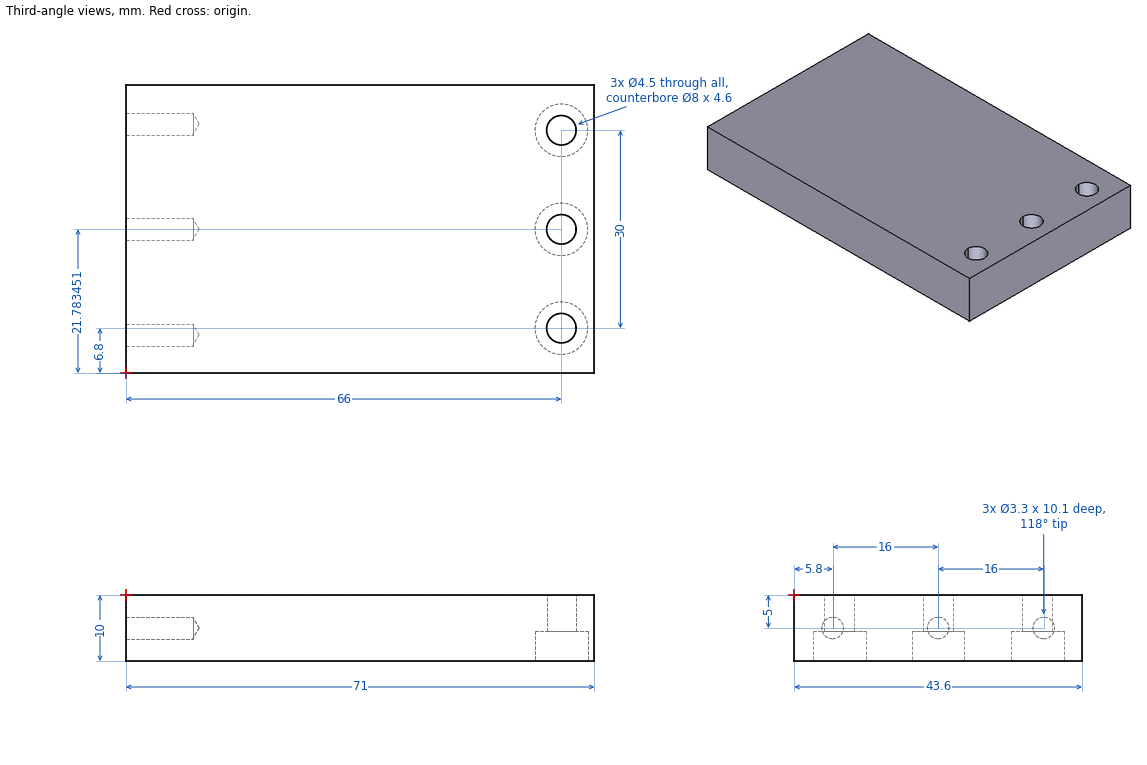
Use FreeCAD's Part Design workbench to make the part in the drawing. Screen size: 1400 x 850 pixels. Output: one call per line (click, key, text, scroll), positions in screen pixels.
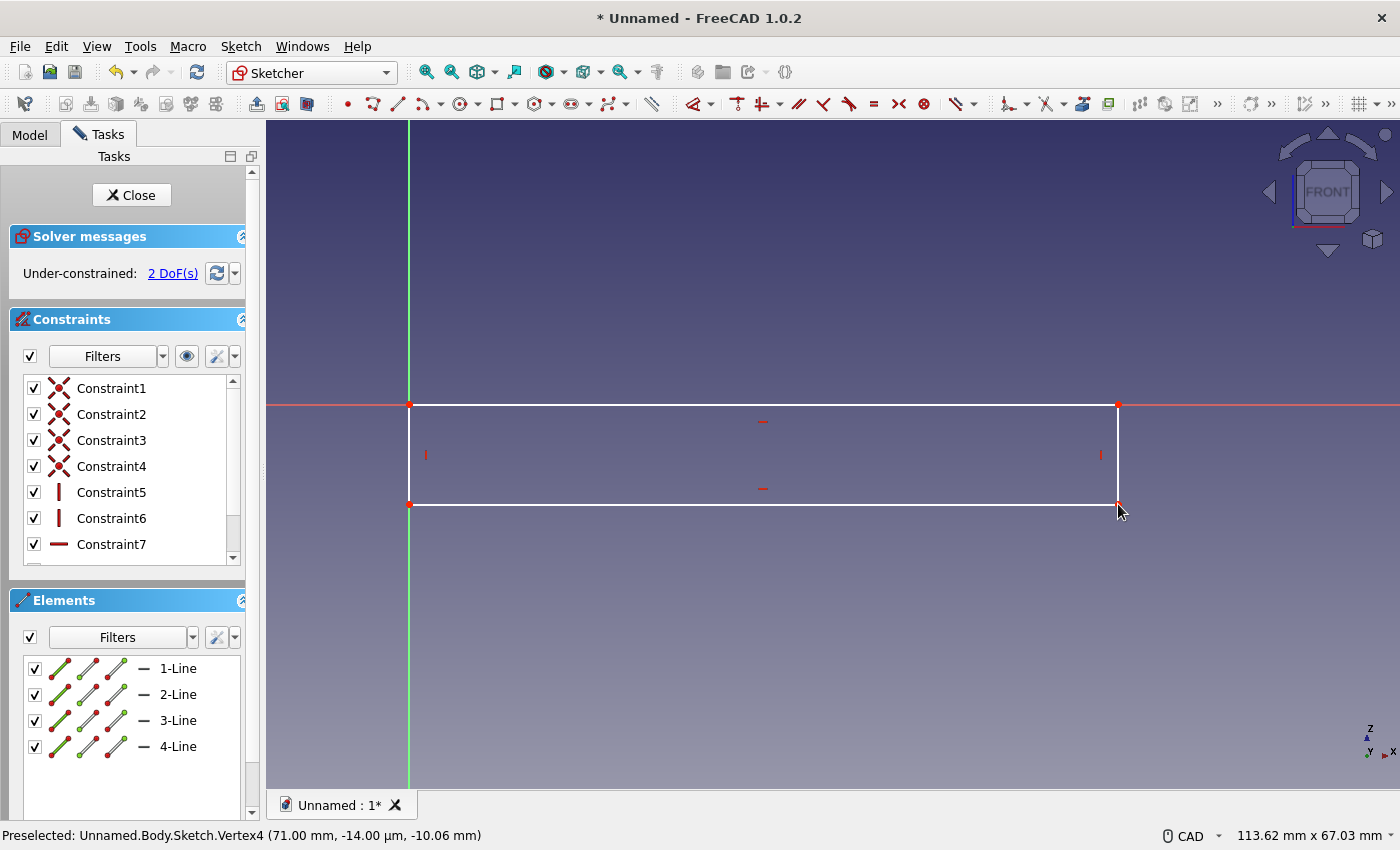
key(d)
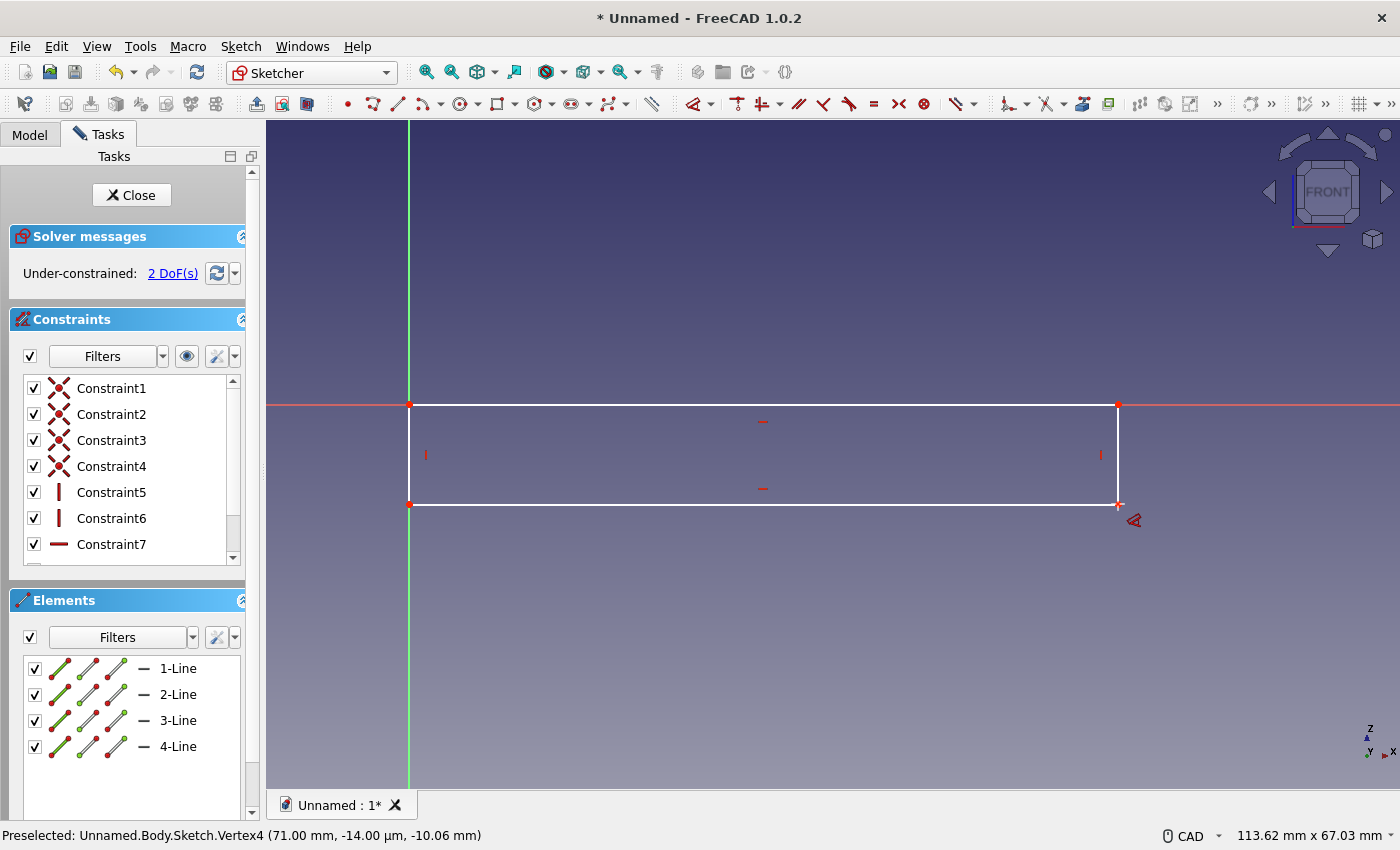
click(409, 435)
click(375, 455)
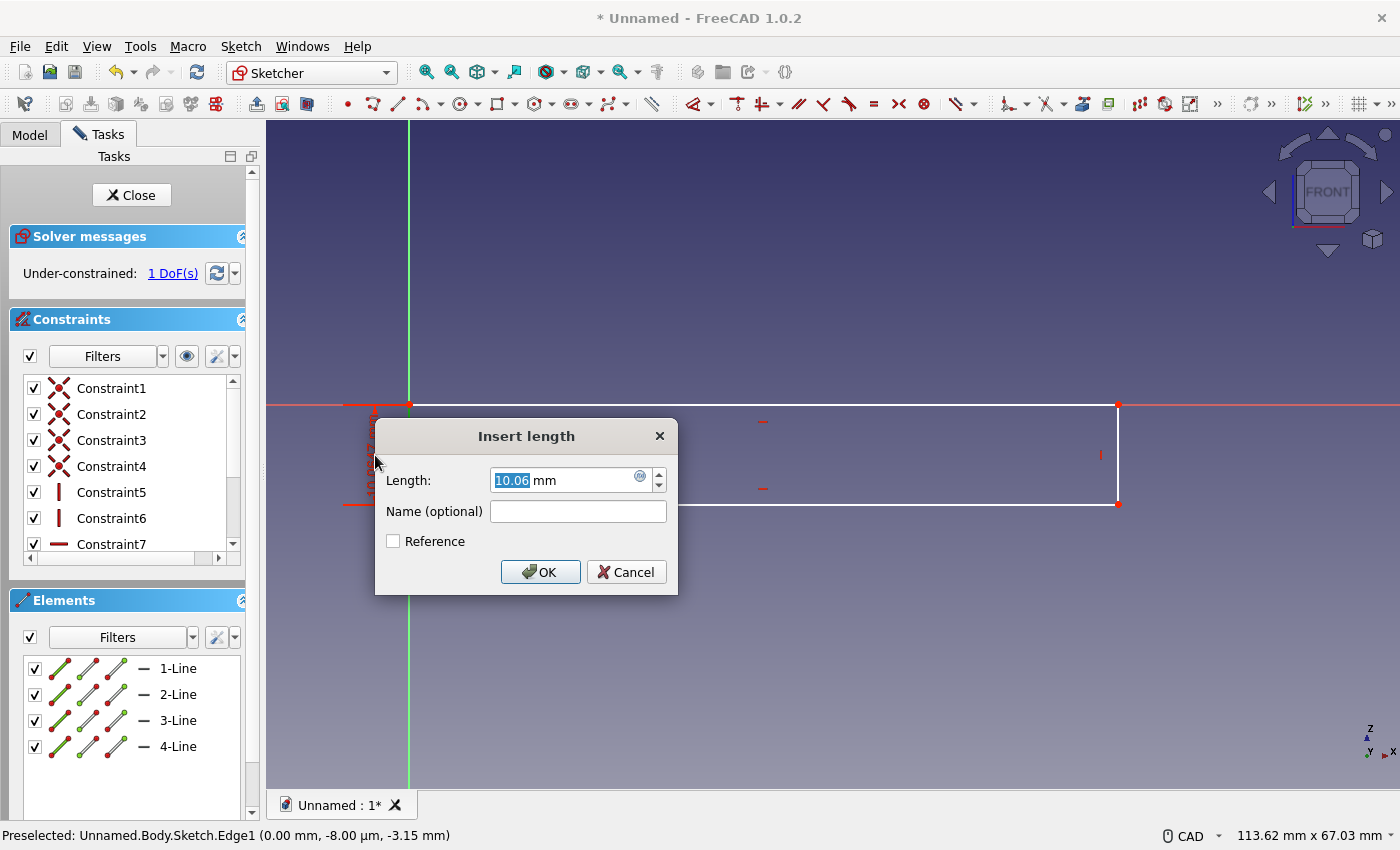
text(10)
key(Return)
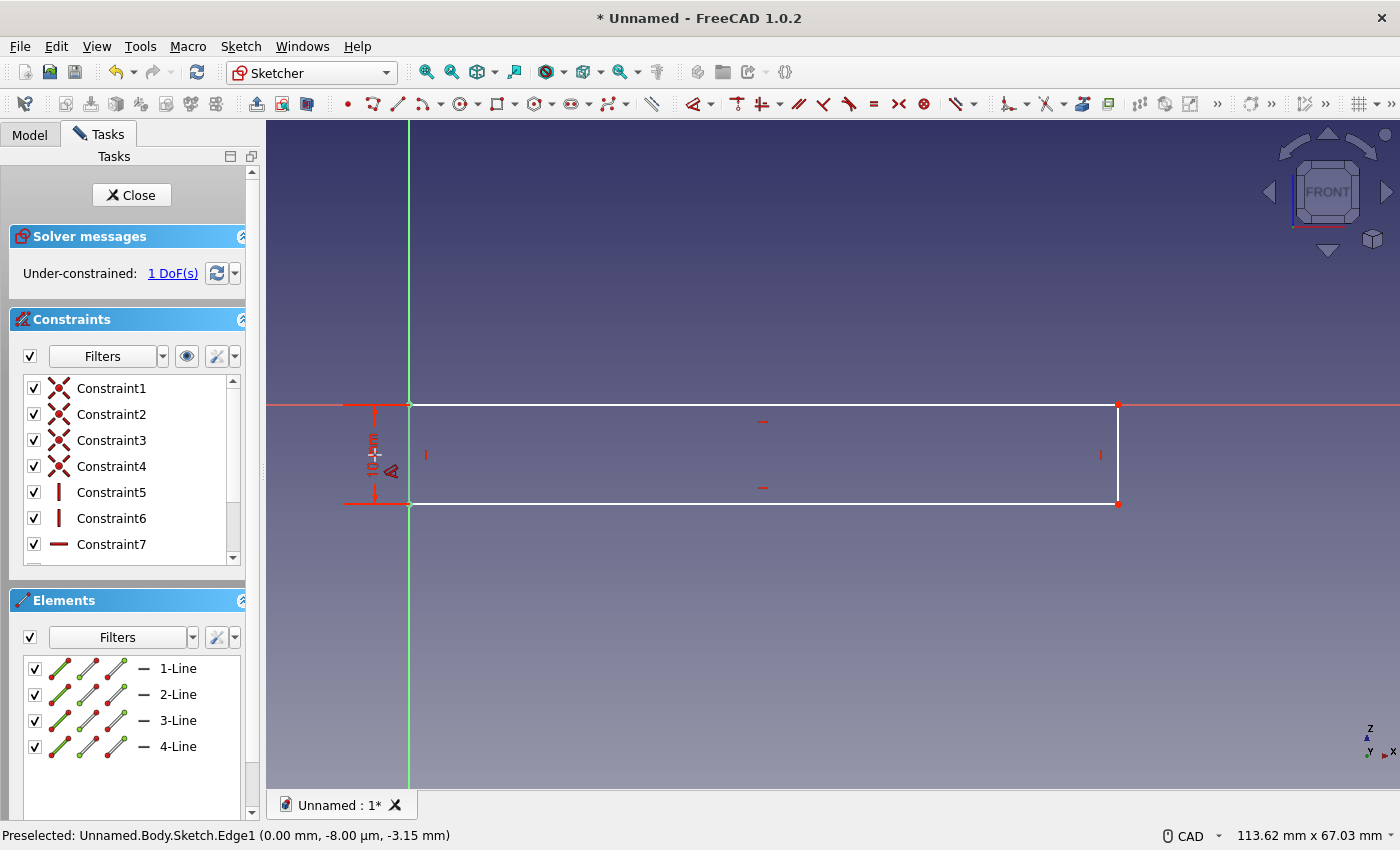
click(622, 504)
click(764, 538)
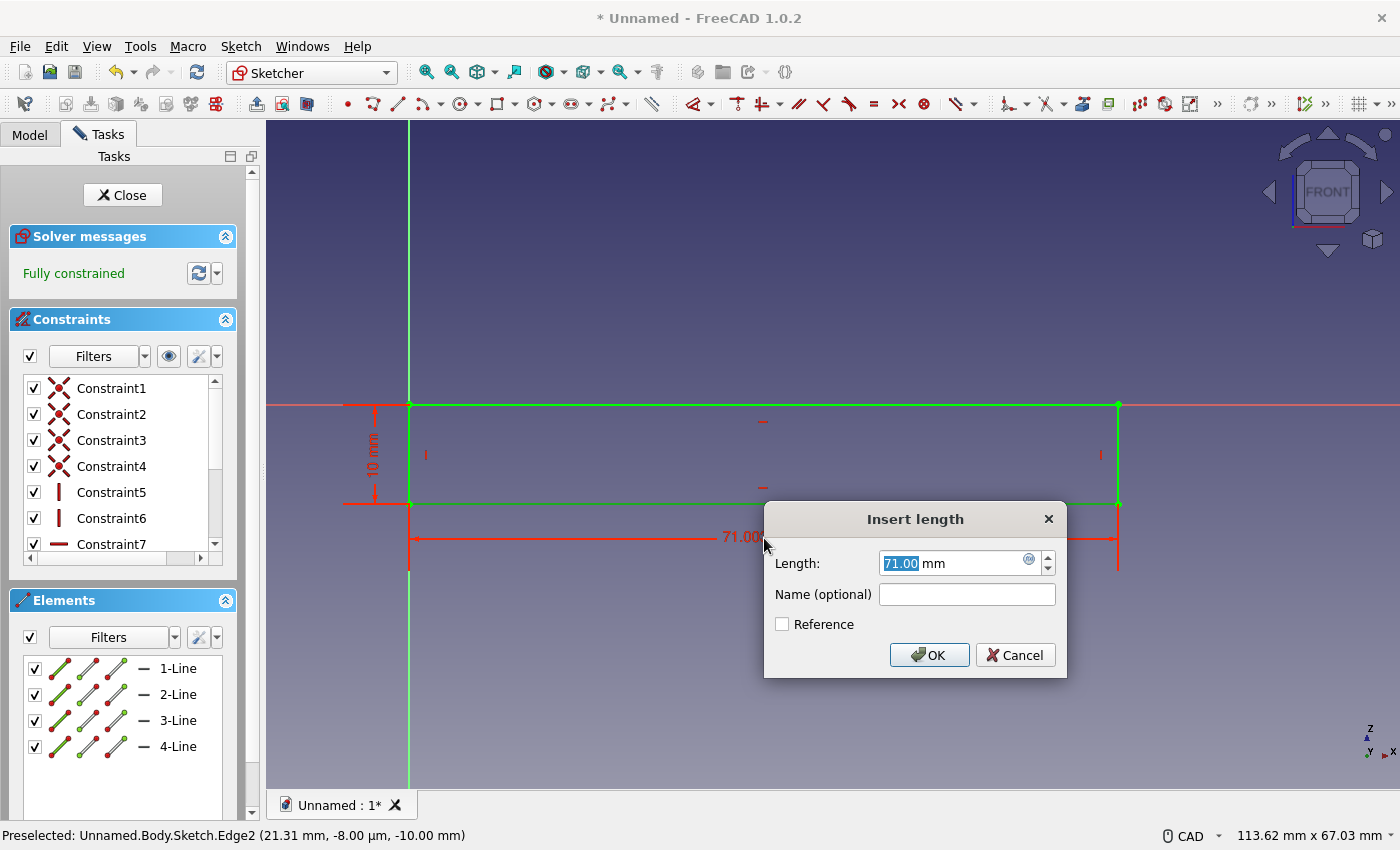
text(71)
key(Return)
key(Escape)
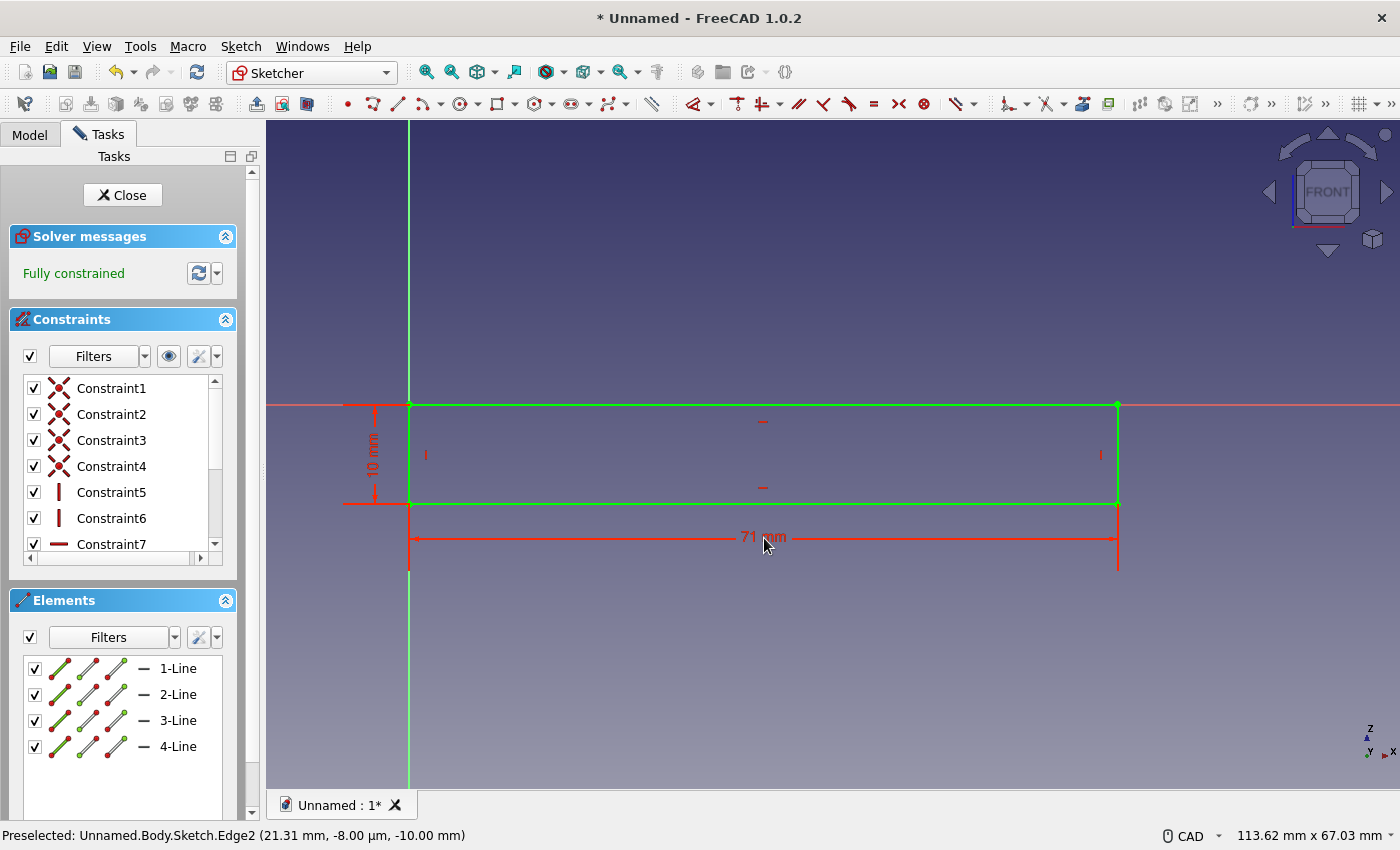
click(123, 195)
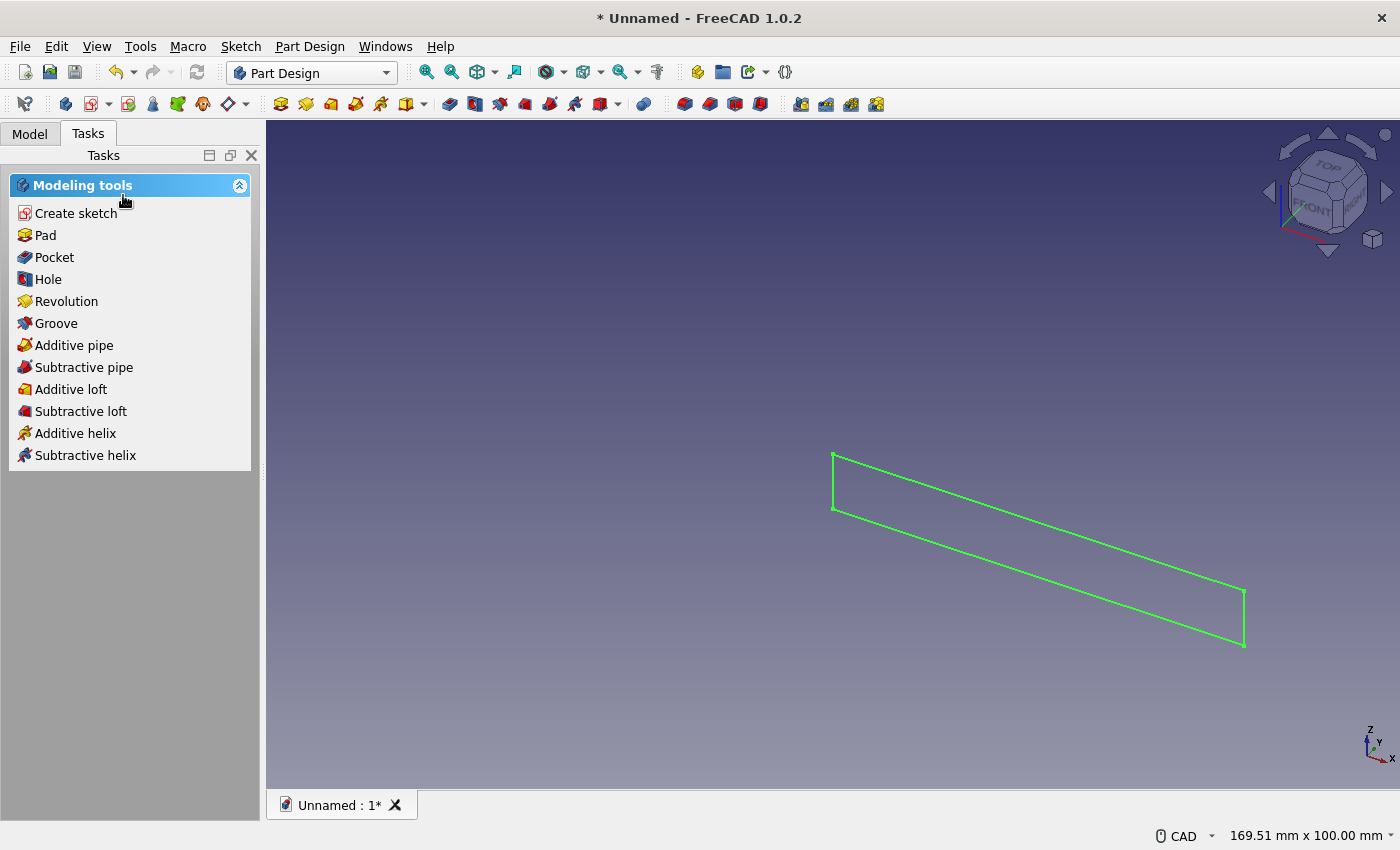
click(281, 104)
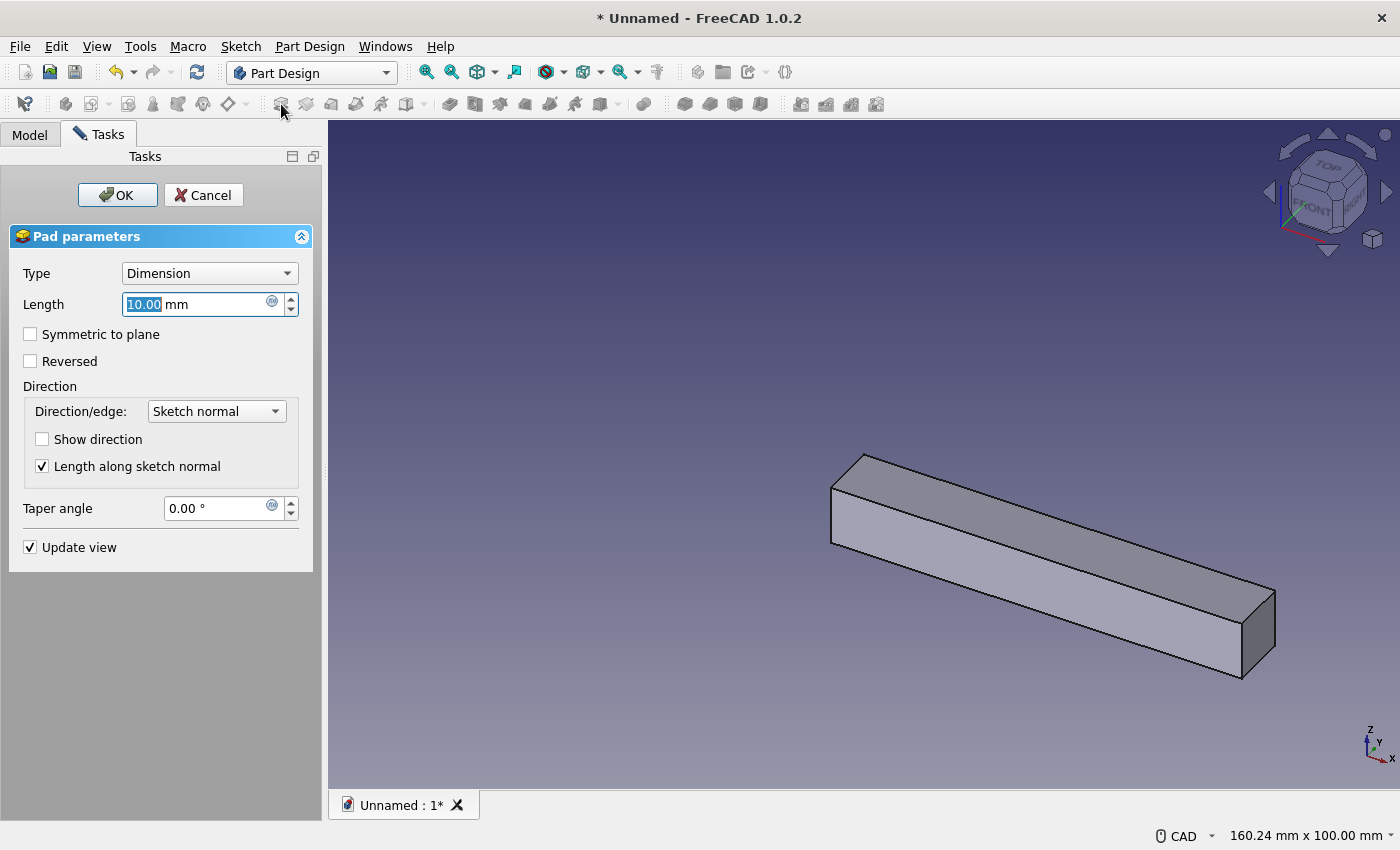
text(43.6)
key(Tab)